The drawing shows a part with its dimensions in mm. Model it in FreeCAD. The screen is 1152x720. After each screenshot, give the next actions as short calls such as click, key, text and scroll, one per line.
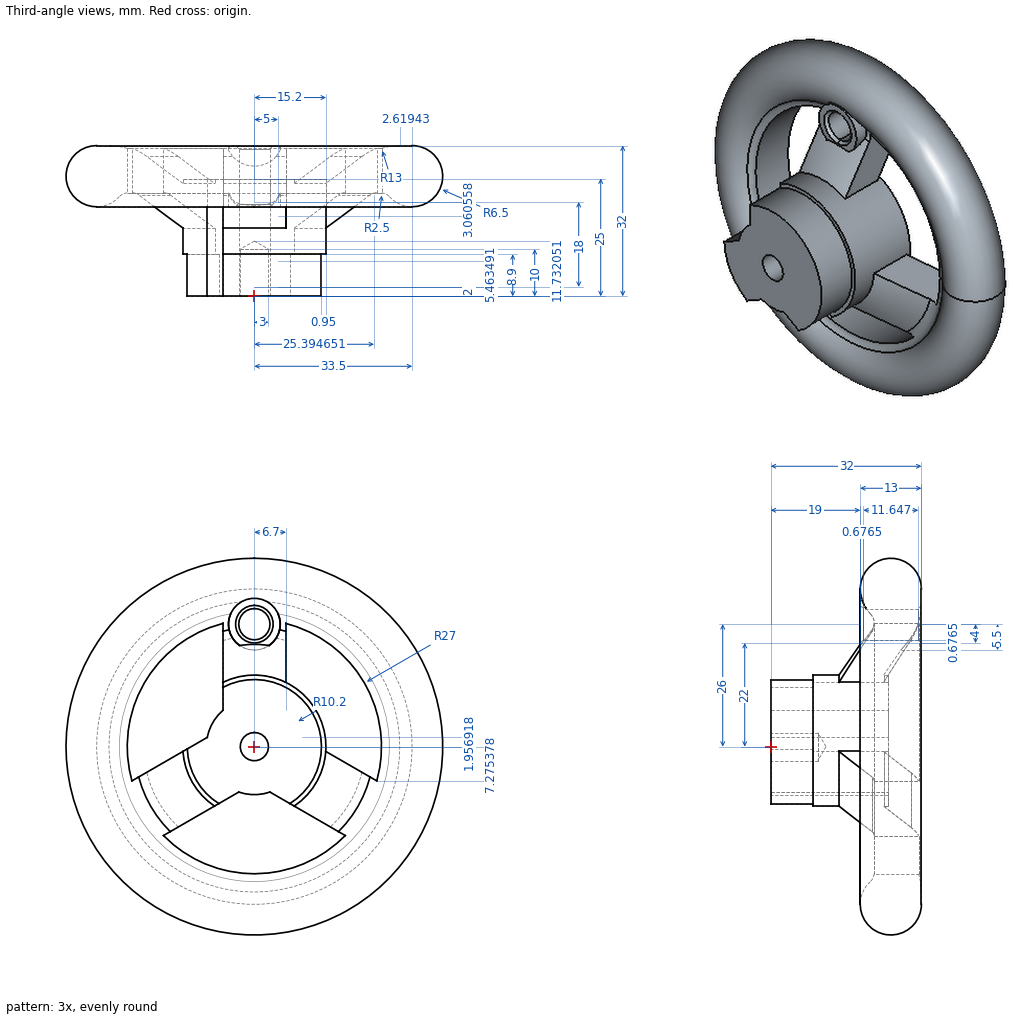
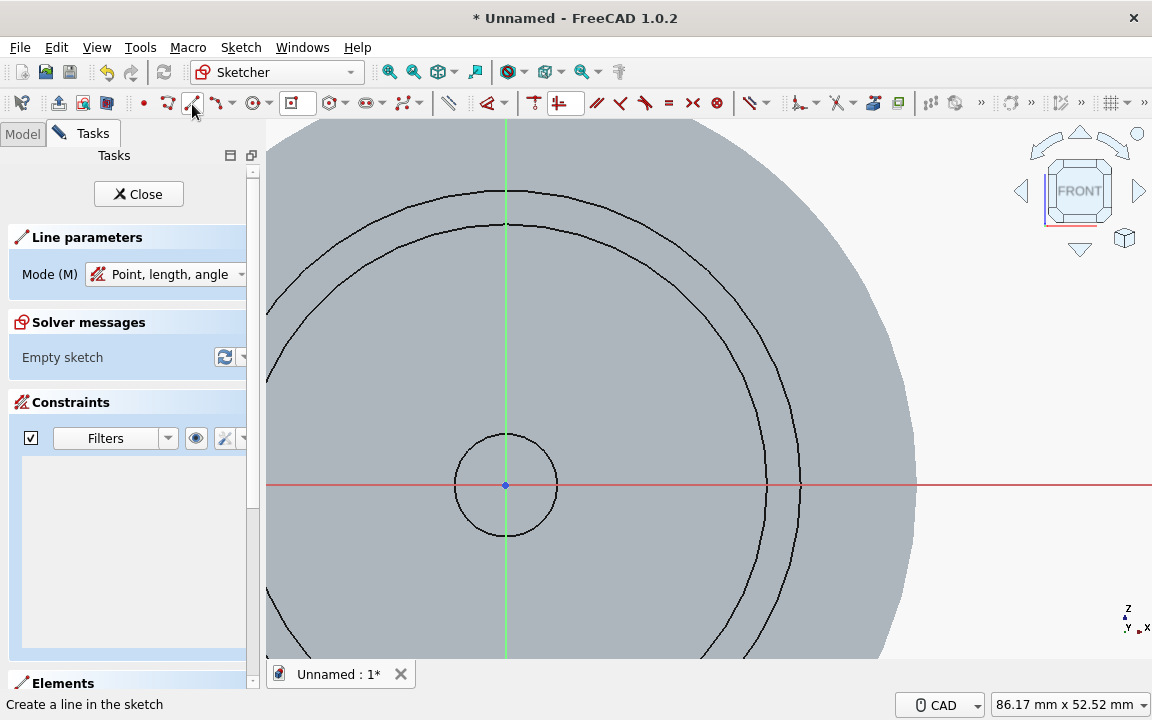
click(773, 560)
click(609, 465)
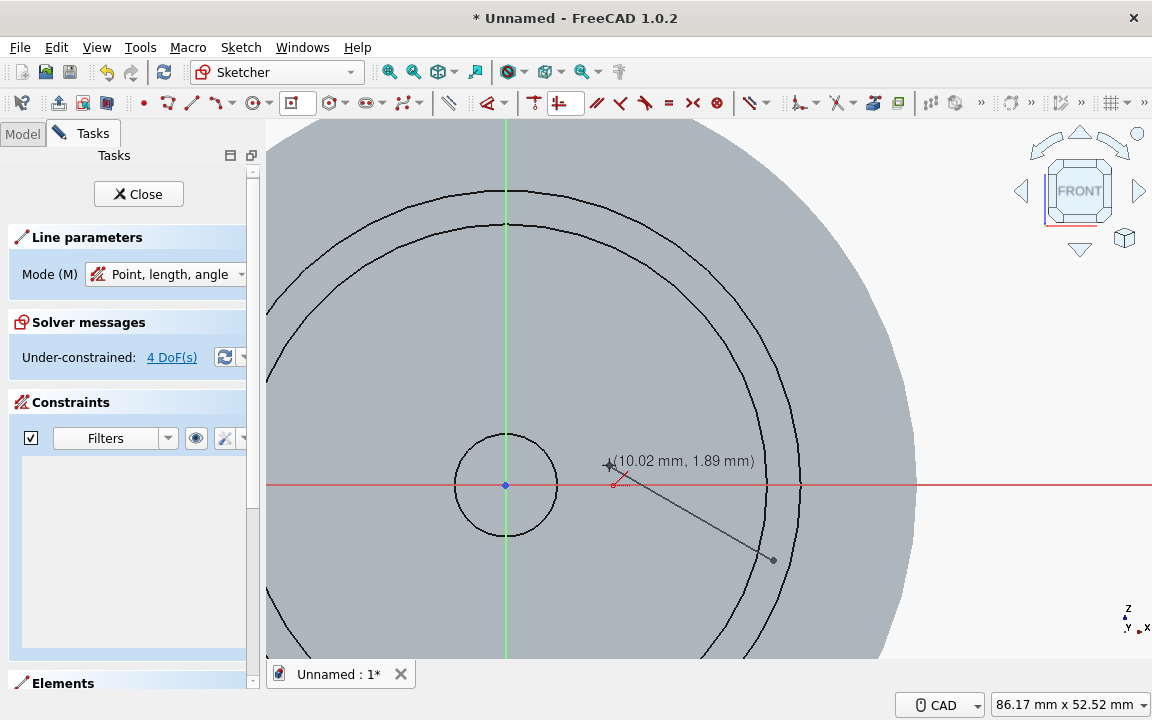
click(575, 406)
click(575, 216)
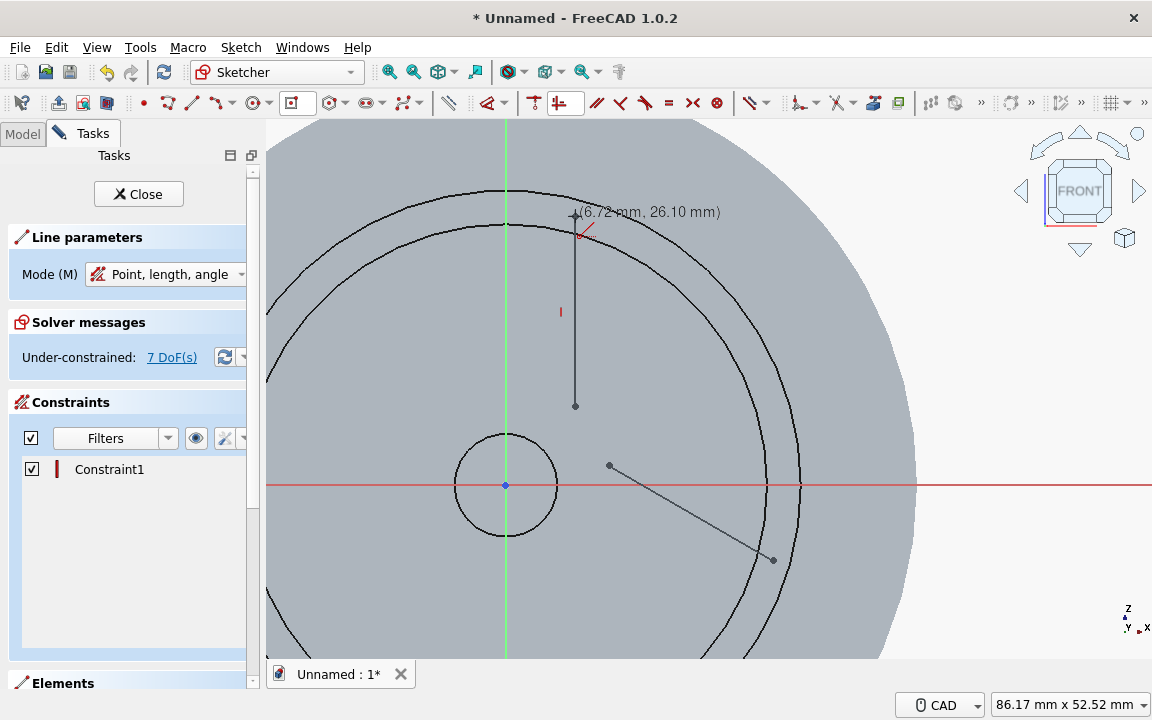
click(216, 104)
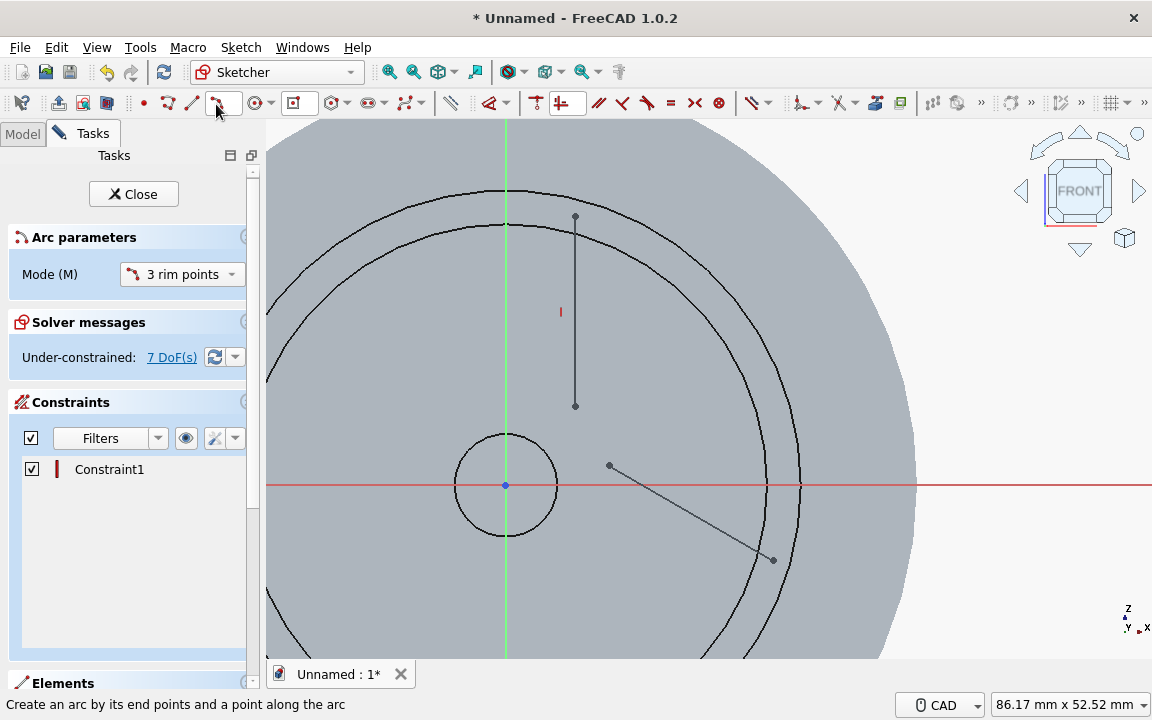
click(609, 466)
click(575, 407)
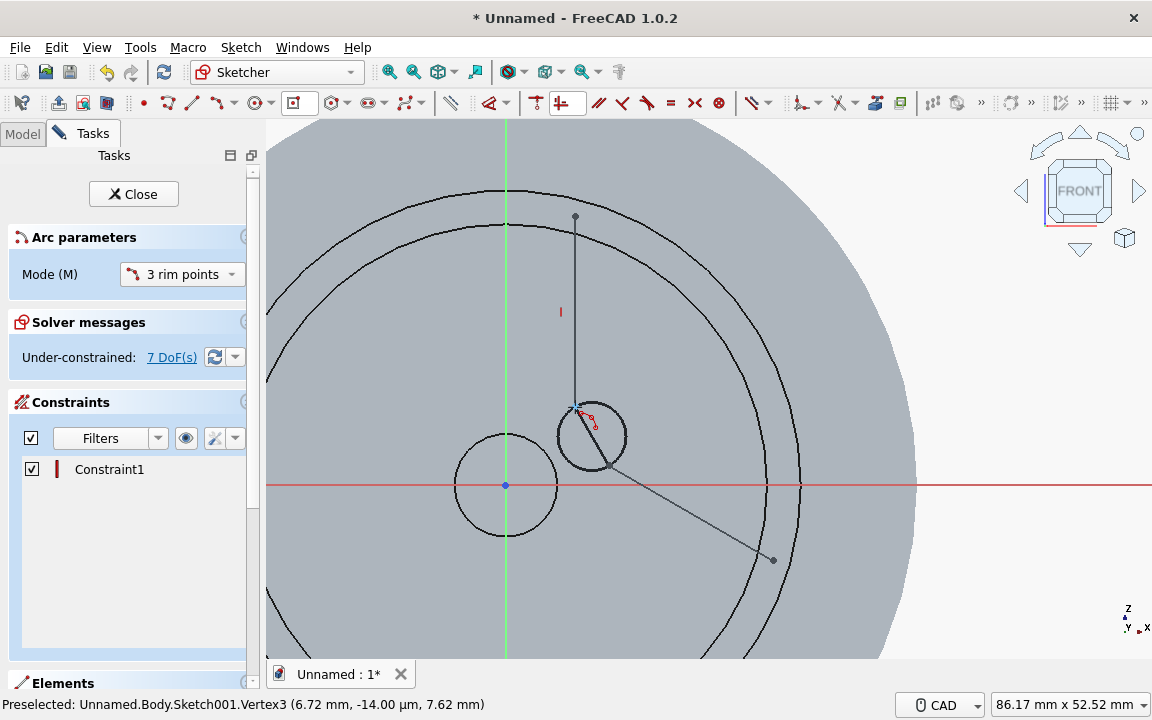
scroll(597, 433, up, 6)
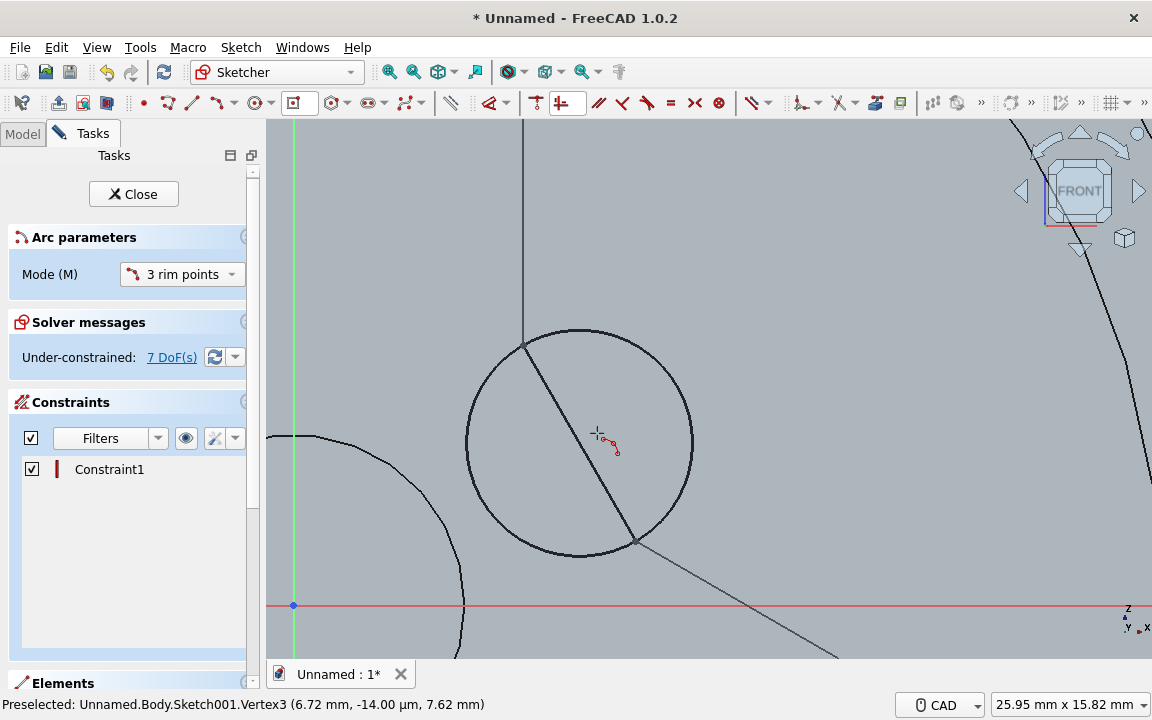
click(595, 431)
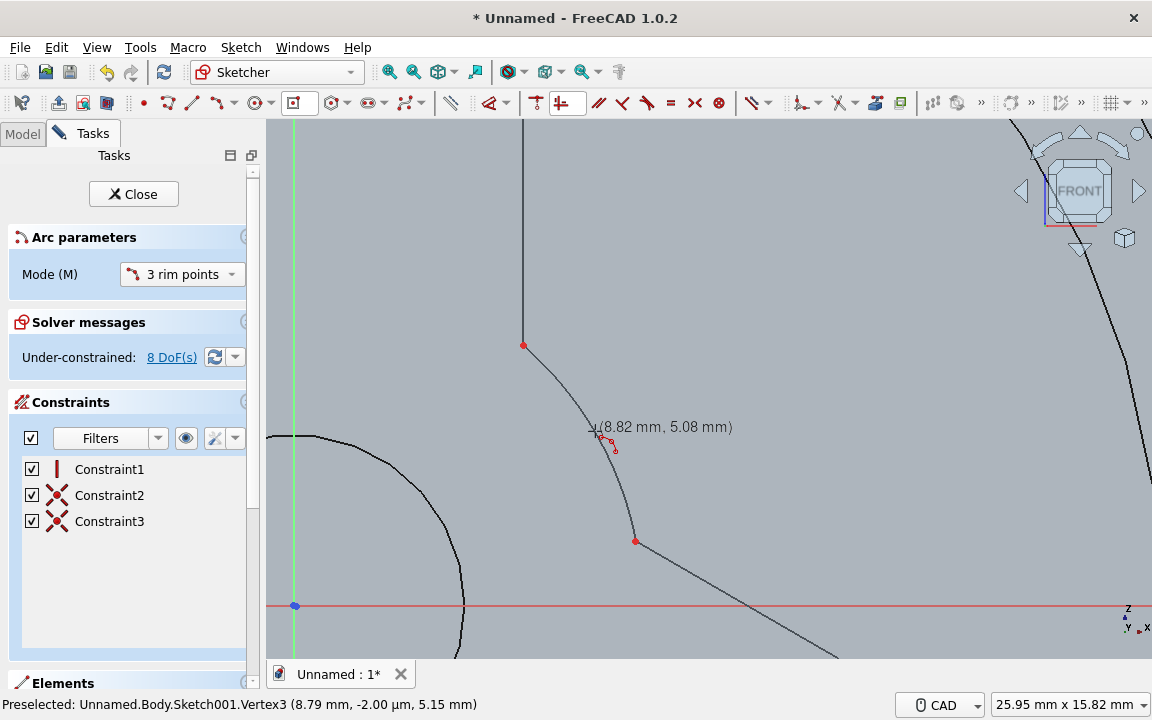
scroll(599, 435, down, 6)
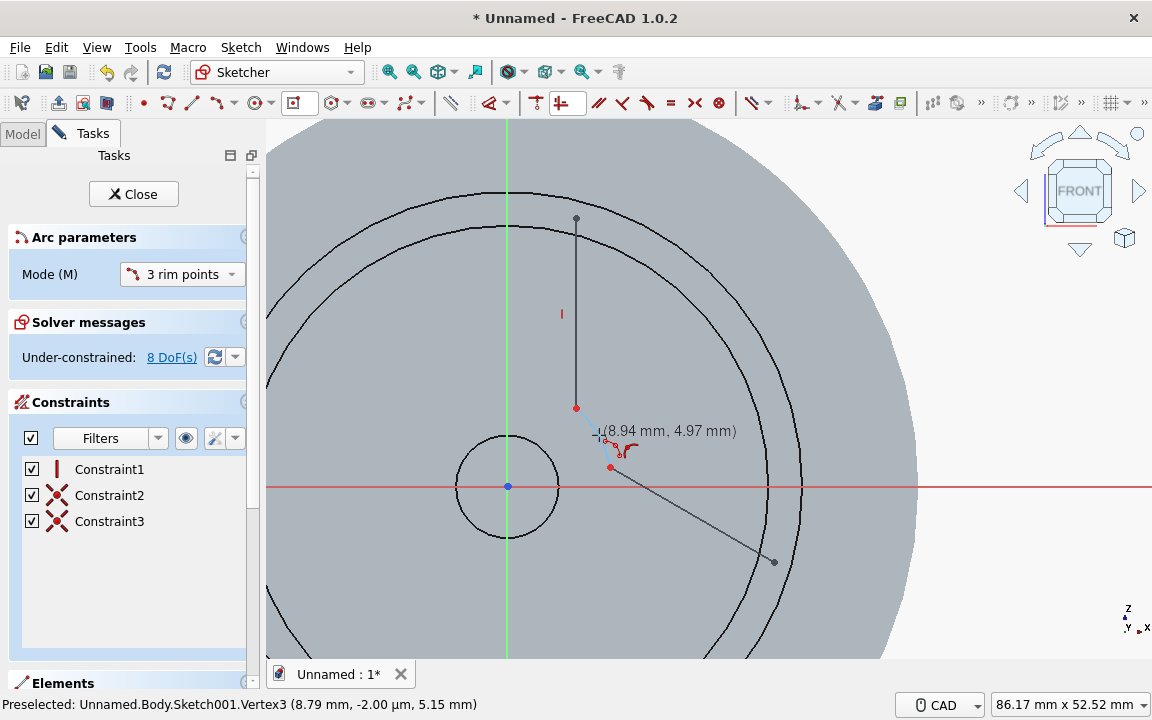
click(576, 218)
click(774, 562)
click(748, 348)
key(Escape)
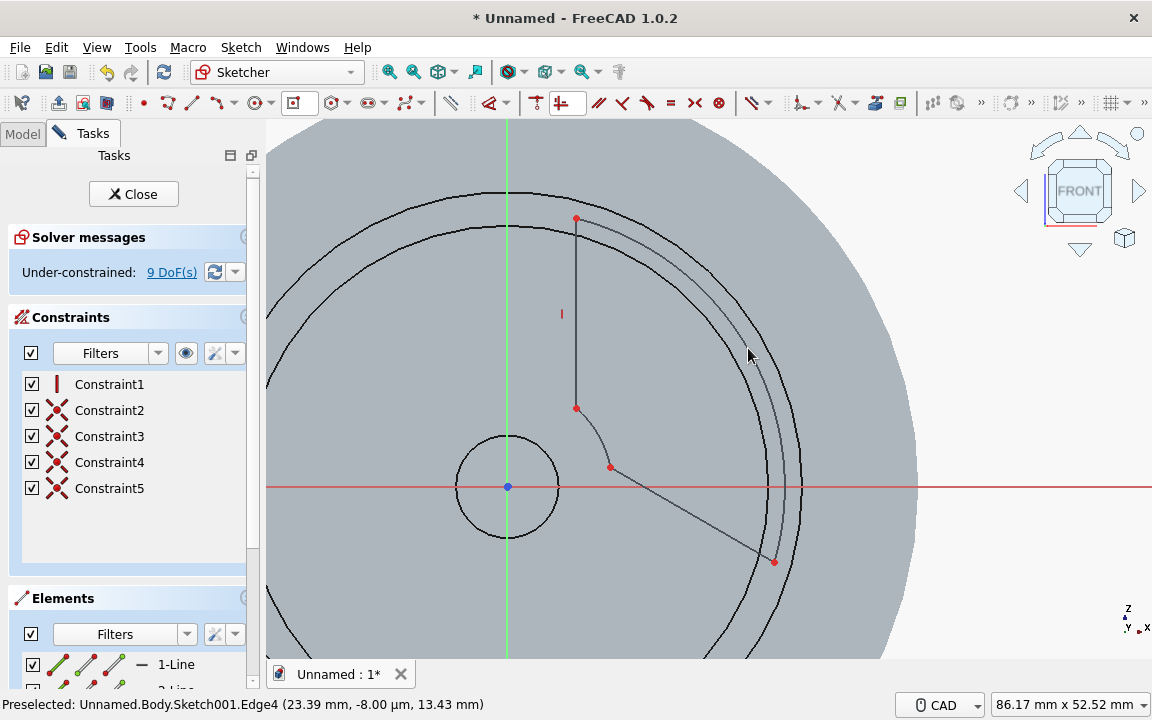
click(604, 447)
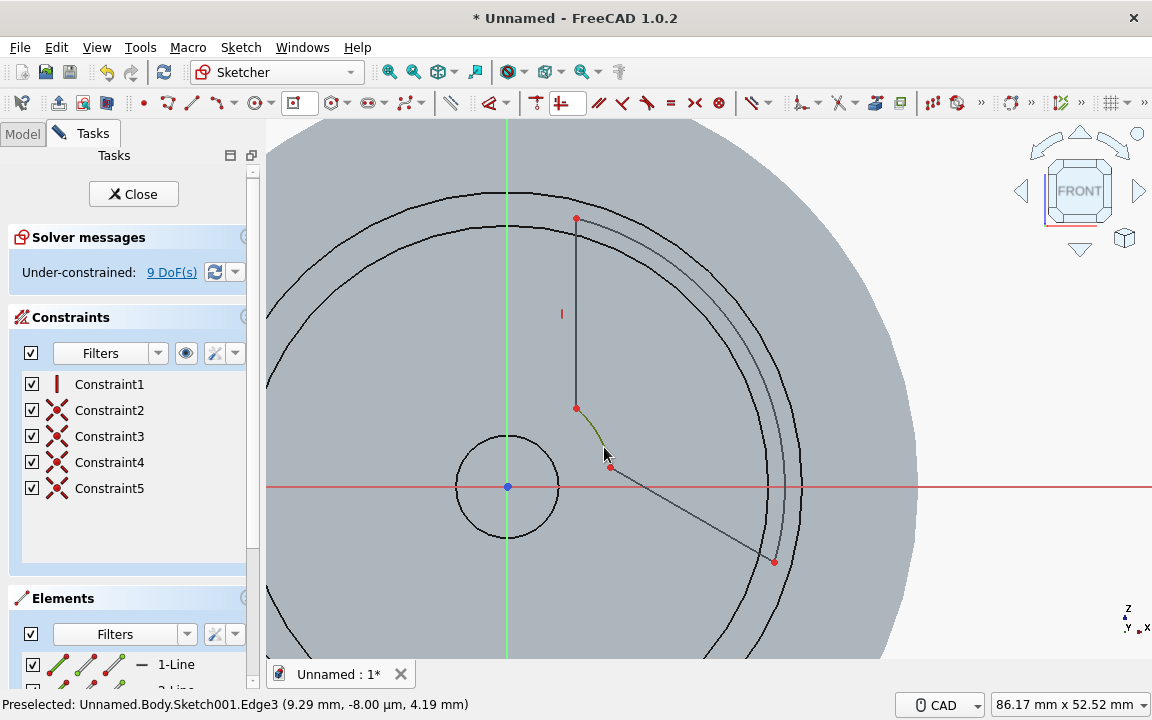
click(779, 431)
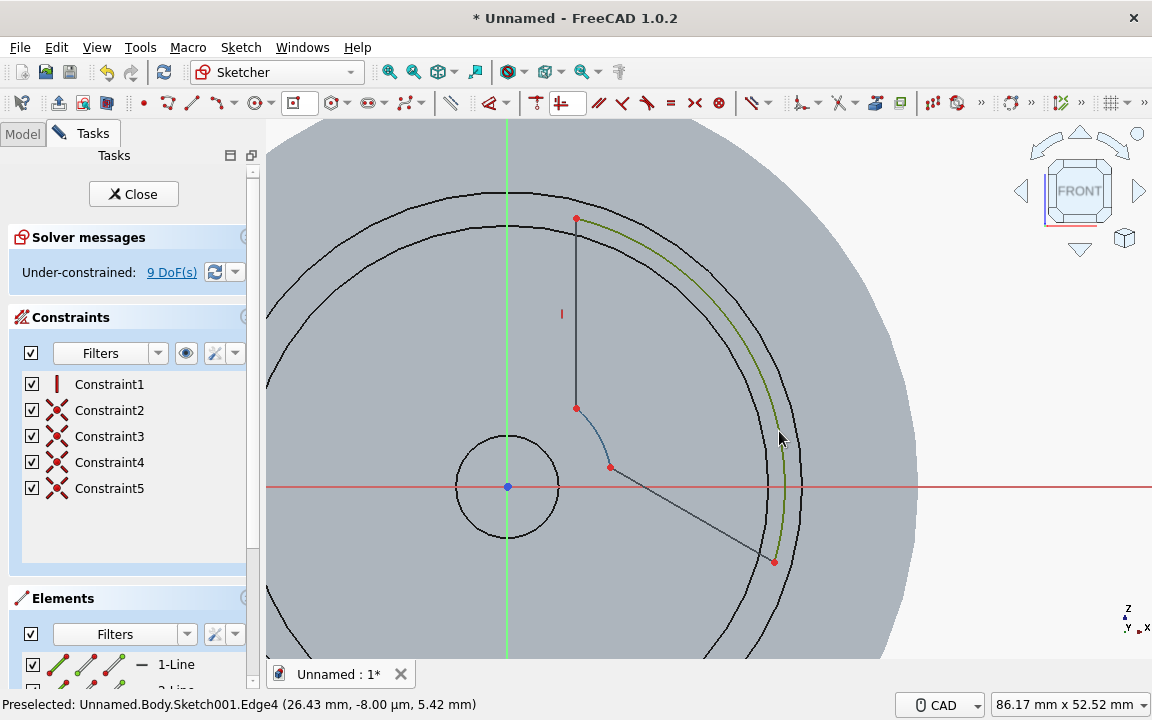
click(536, 104)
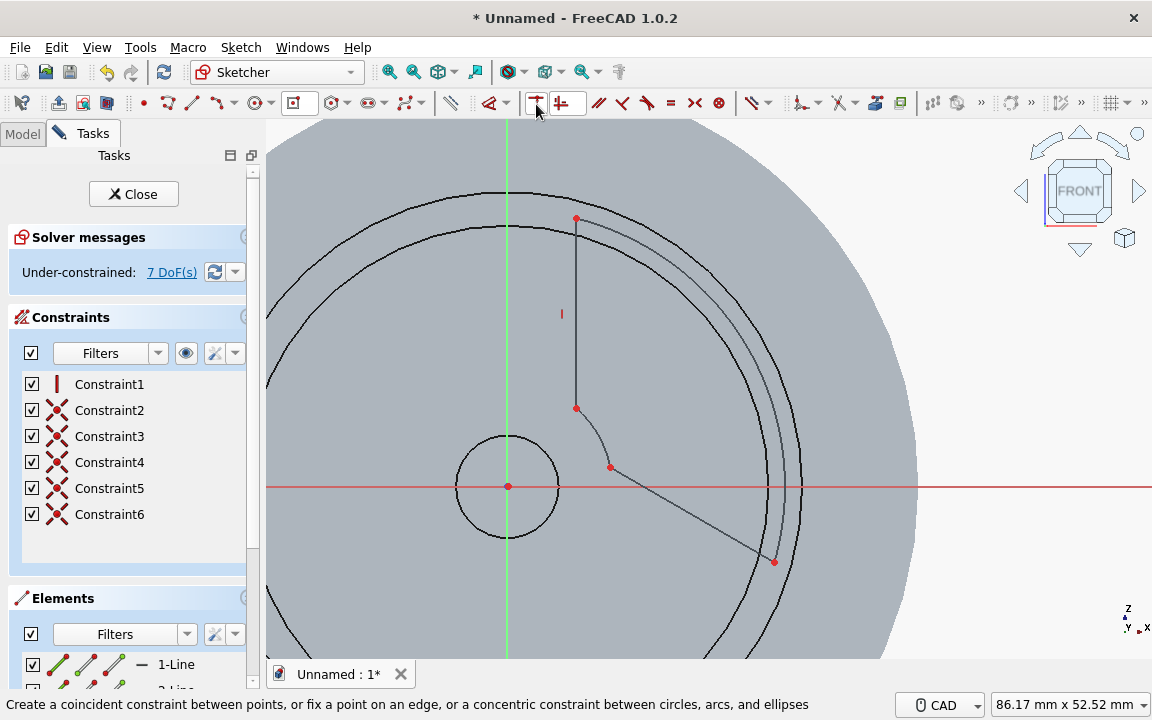
drag(497, 477, 518, 497)